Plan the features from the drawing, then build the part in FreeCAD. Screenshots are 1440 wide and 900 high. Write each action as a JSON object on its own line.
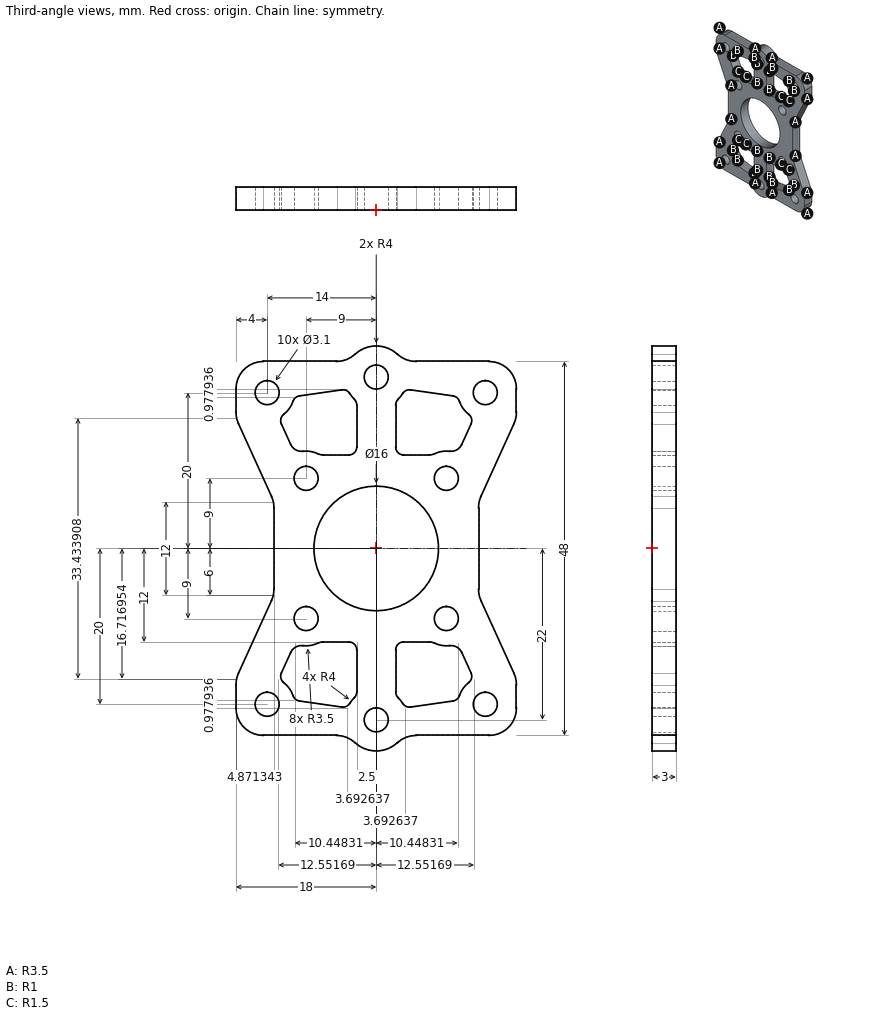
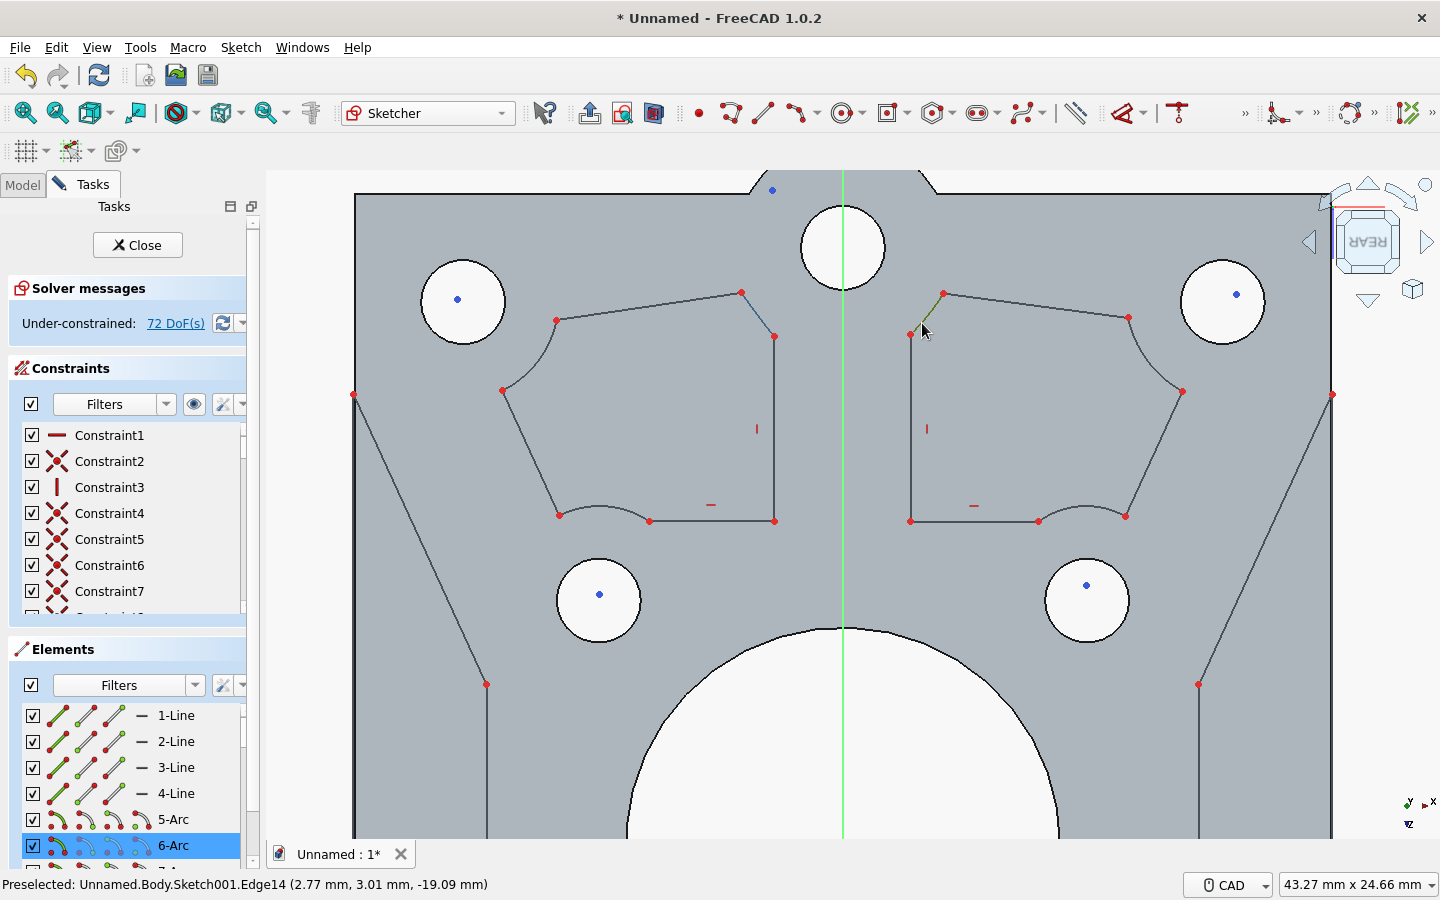
{"action": "left_click", "coordinate": [1178, 114]}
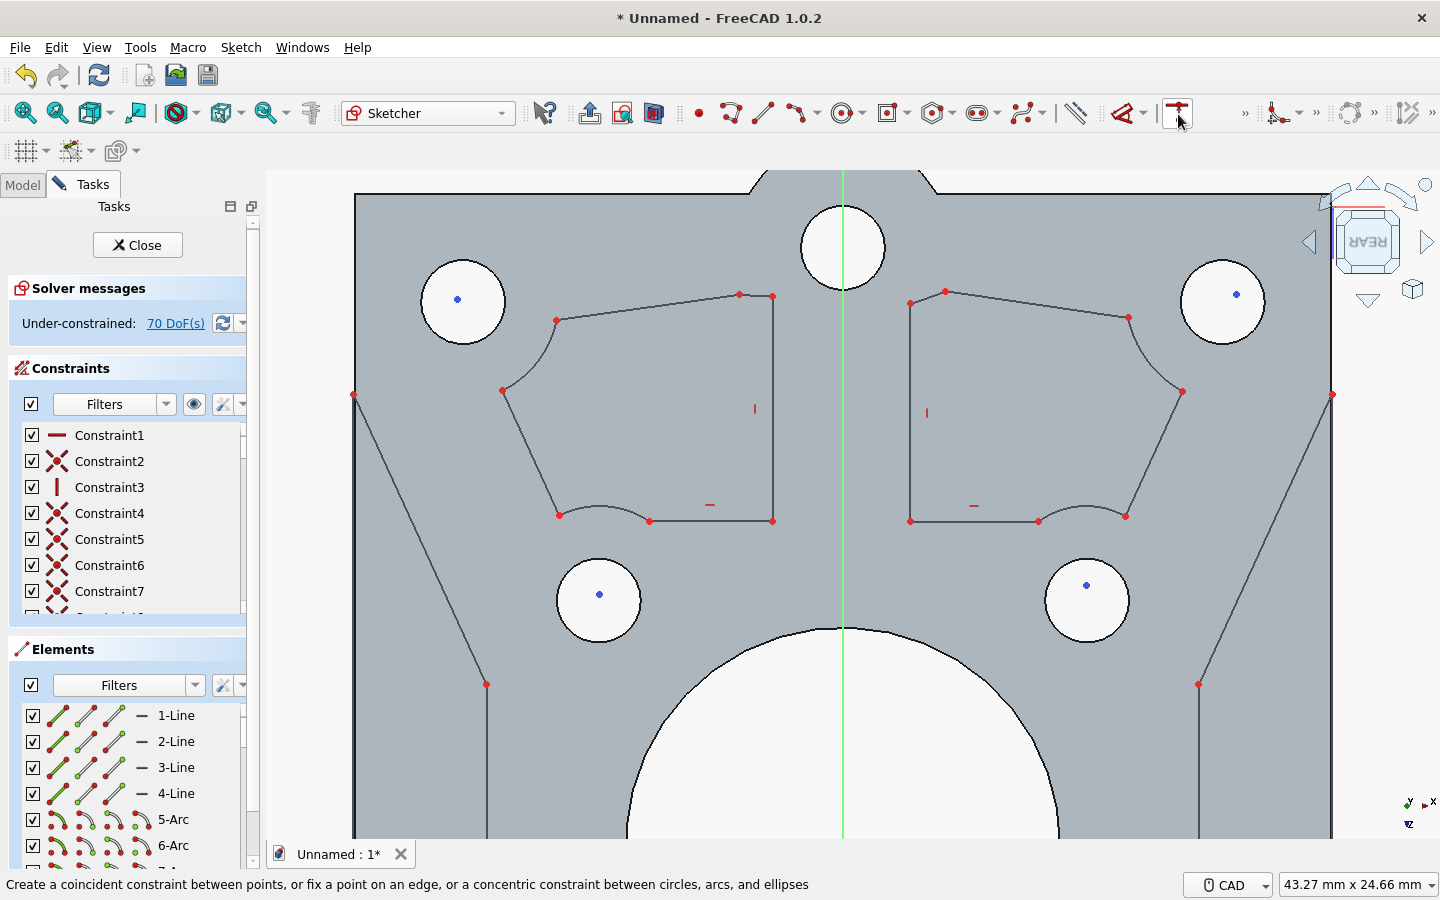
{"action": "scroll", "coordinate": [750, 307], "scroll_direction": "down", "scroll_amount": 5}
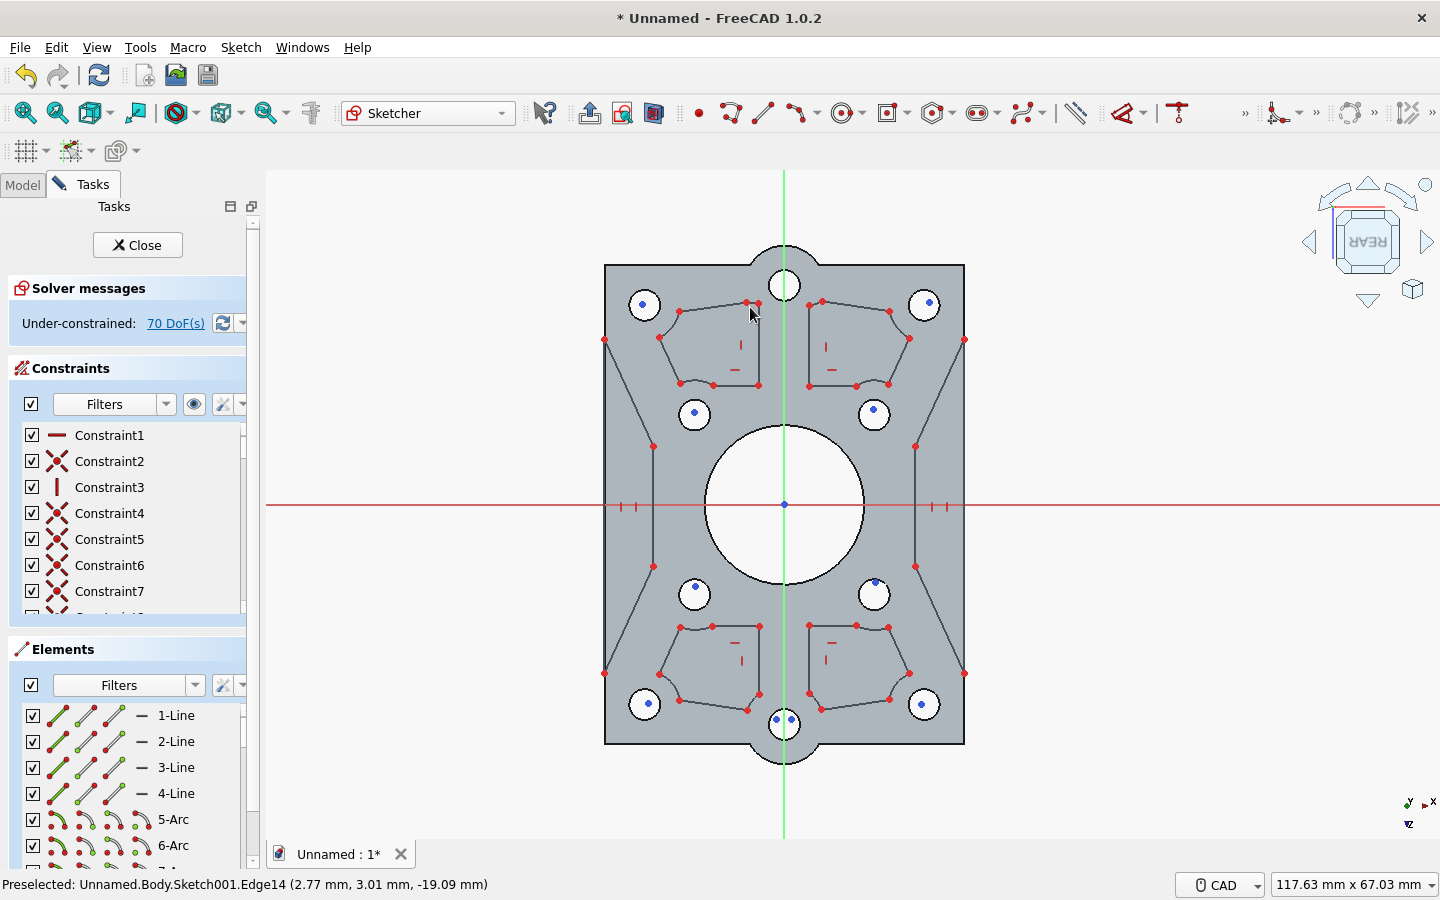
{"action": "scroll", "coordinate": [755, 698], "scroll_direction": "up", "scroll_amount": 5}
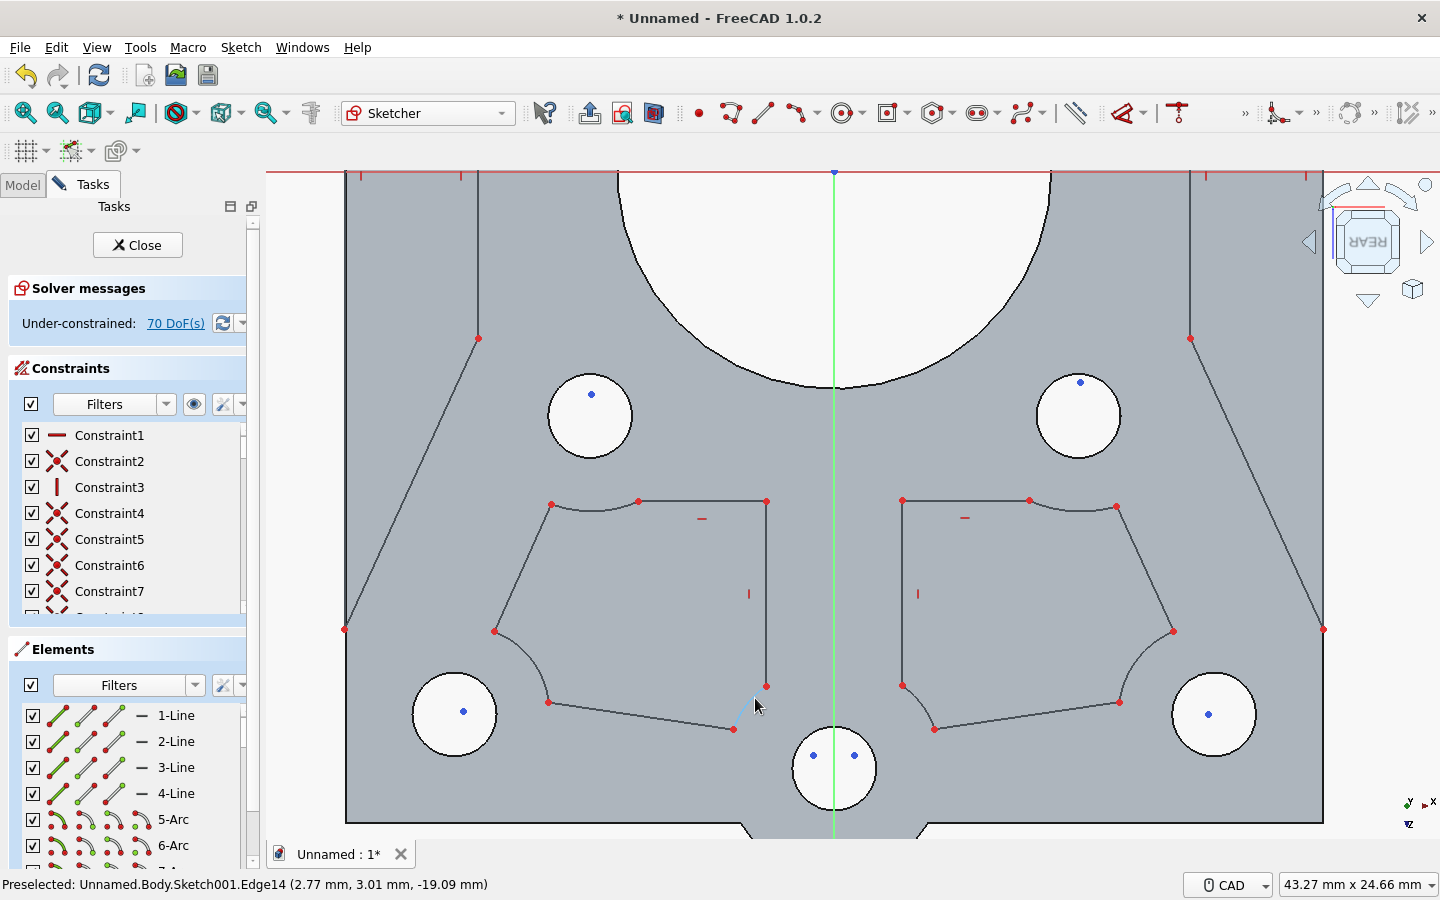
{"action": "left_click", "coordinate": [753, 697]}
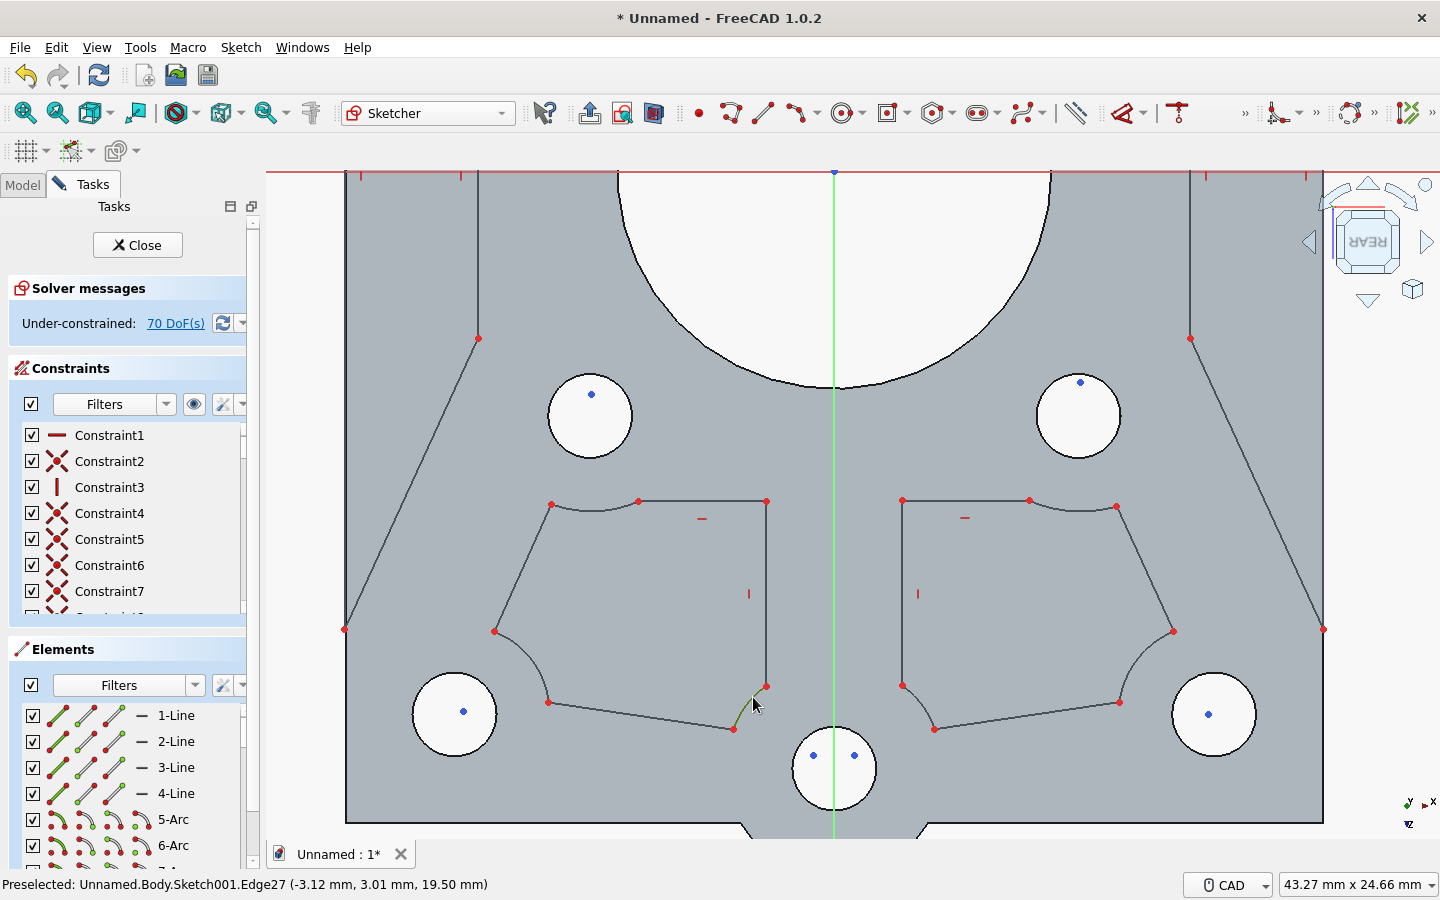
{"action": "left_click", "coordinate": [928, 714]}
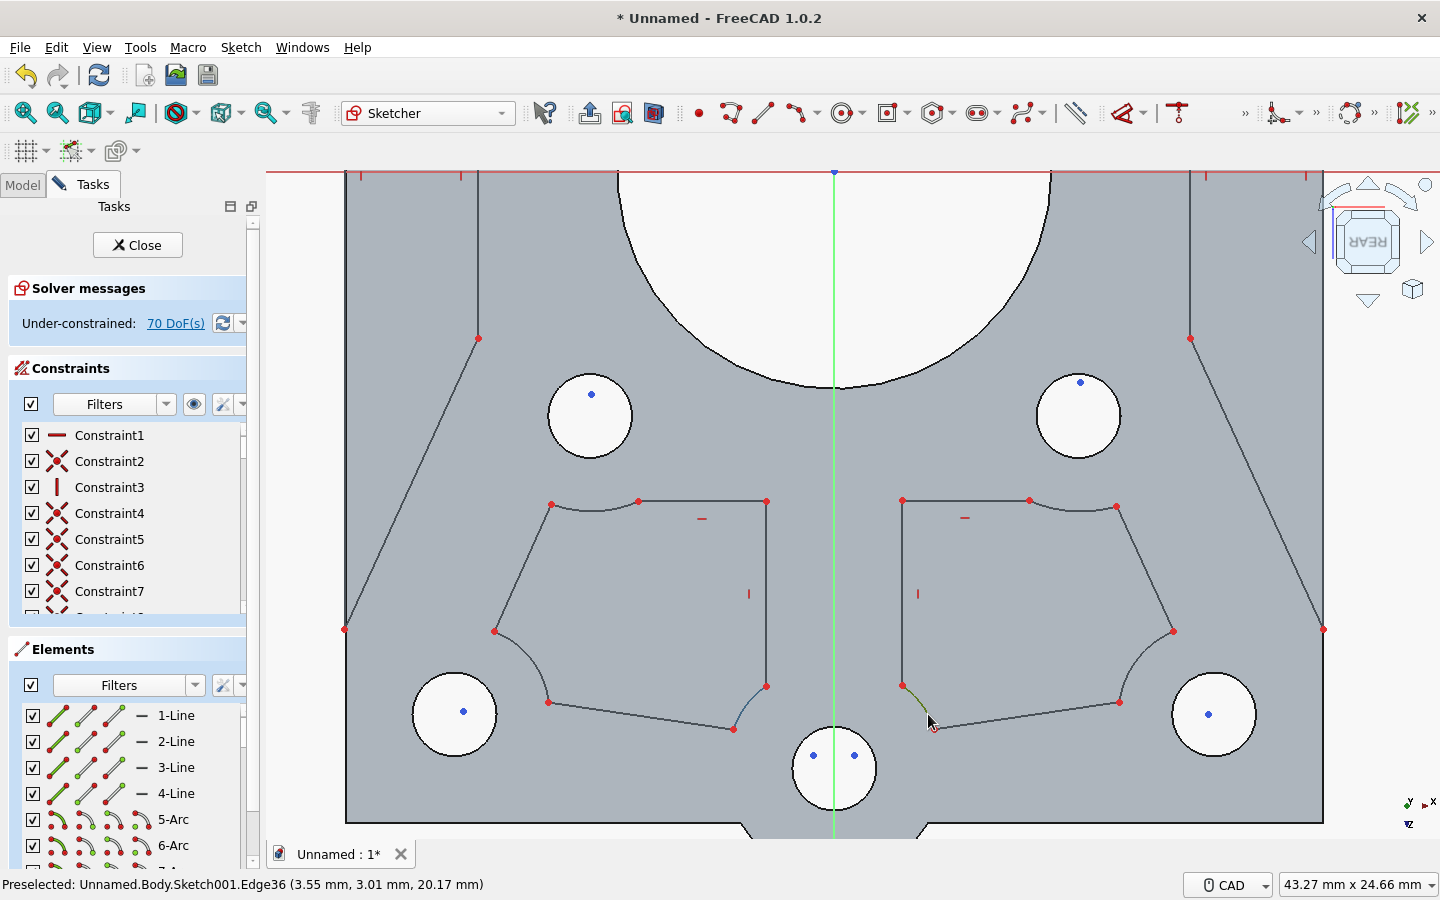
{"action": "left_click", "coordinate": [1178, 114]}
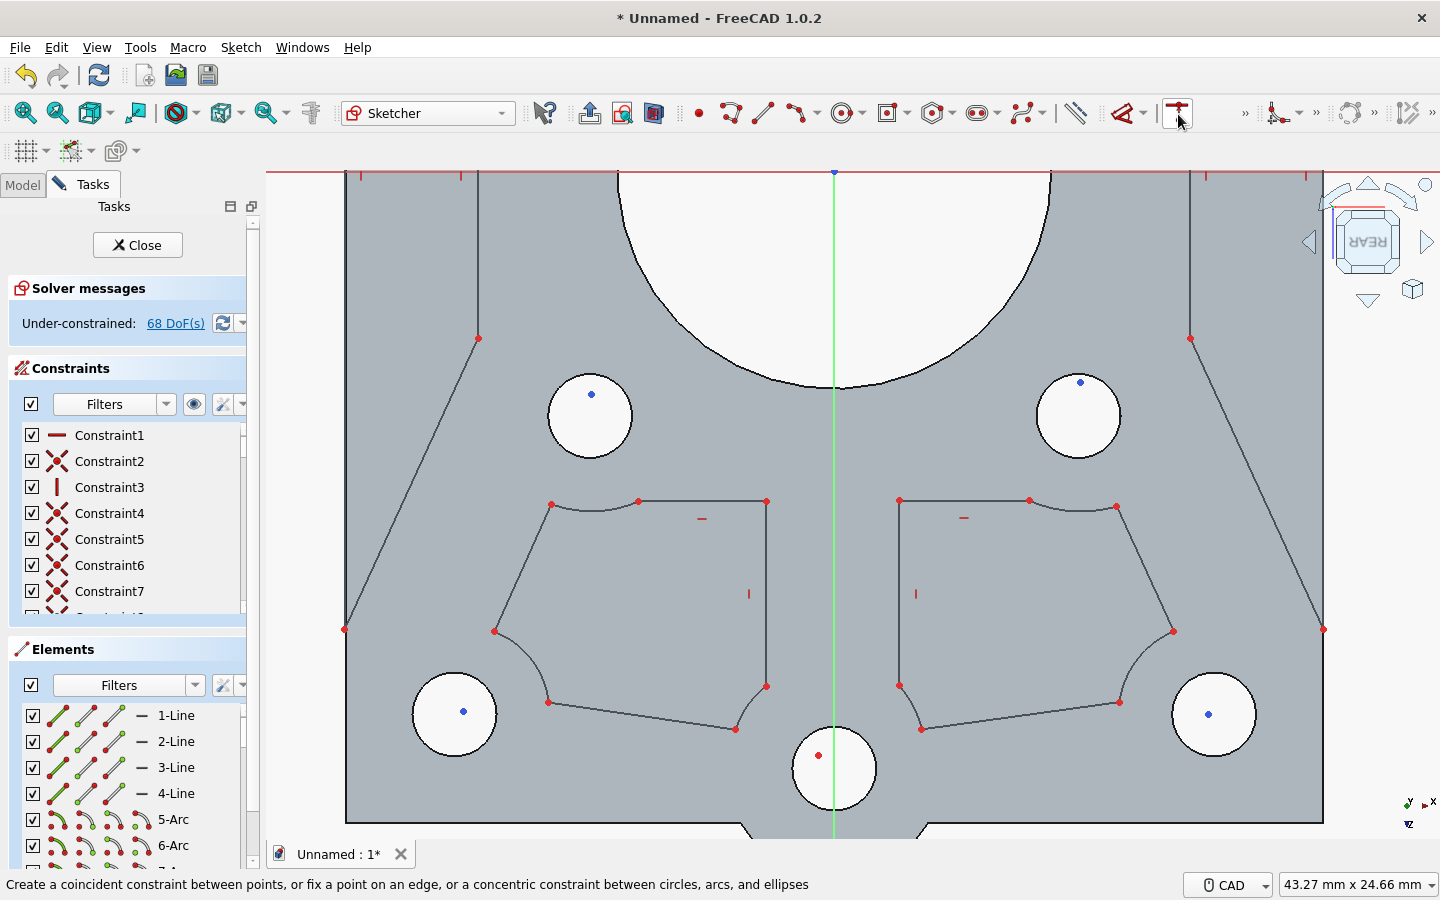
{"action": "scroll", "coordinate": [755, 698], "scroll_direction": "down", "scroll_amount": 5}